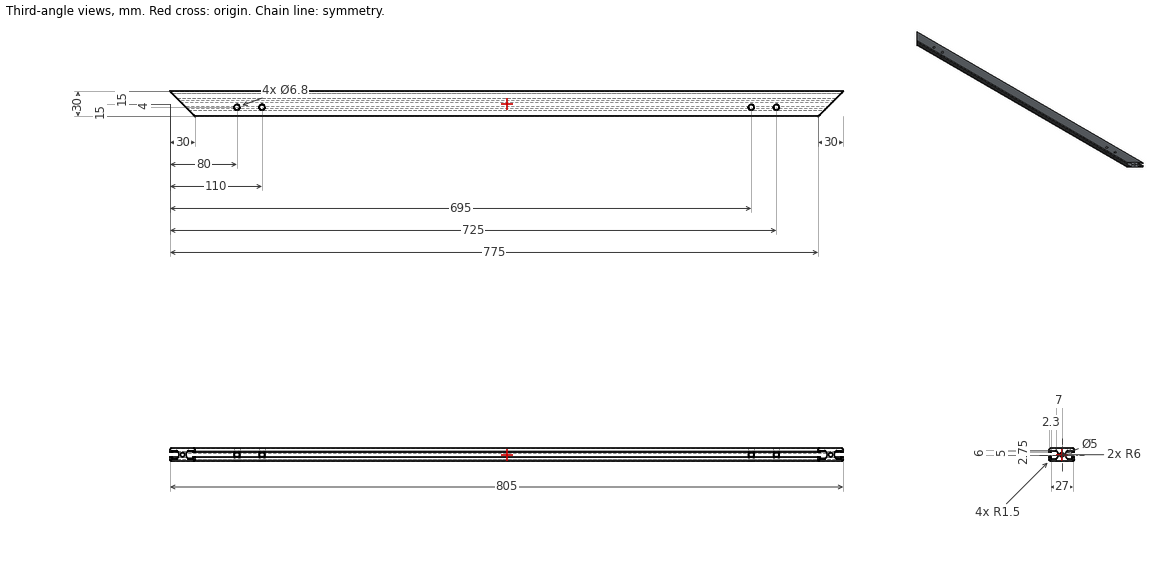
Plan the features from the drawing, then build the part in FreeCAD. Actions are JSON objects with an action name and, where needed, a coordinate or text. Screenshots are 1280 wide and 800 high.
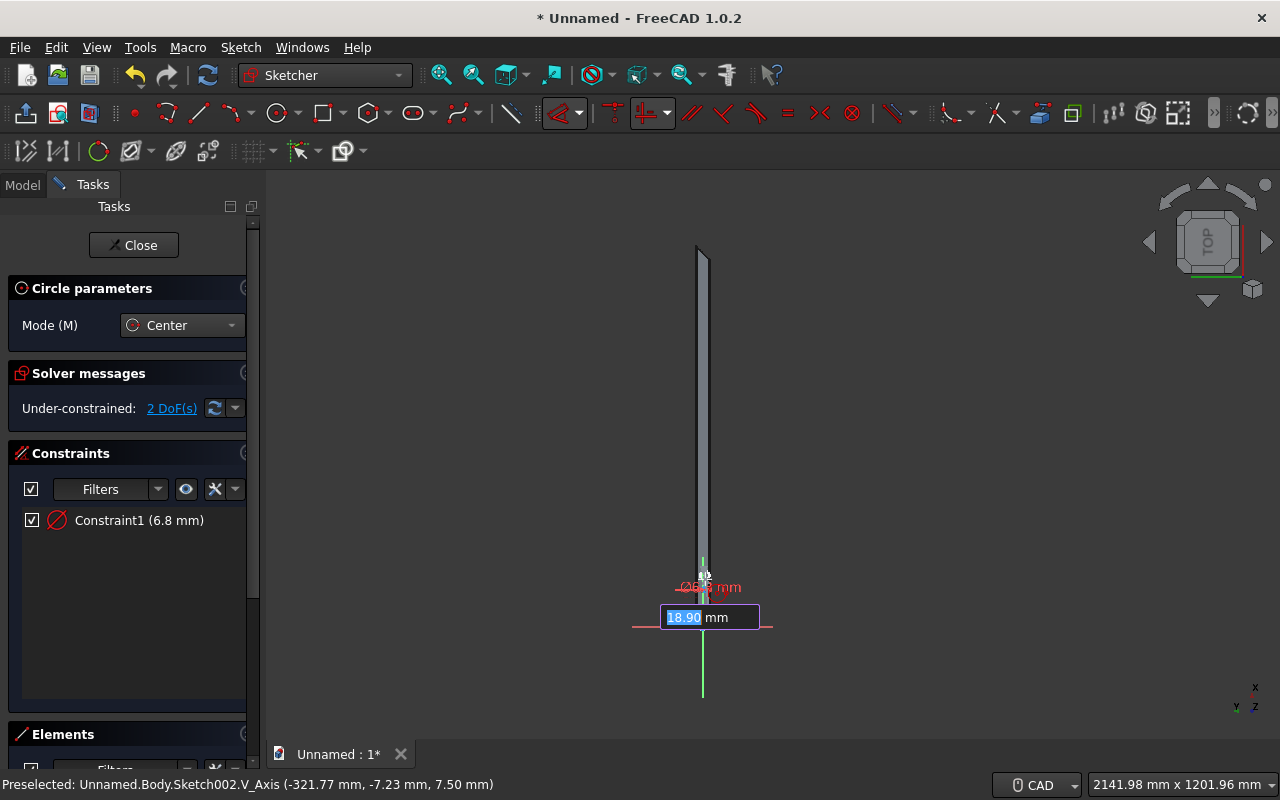
{"action": "scroll", "coordinate": [706, 574], "scroll_direction": "up", "scroll_amount": 9}
{"action": "mouse_move", "coordinate": [704, 571]}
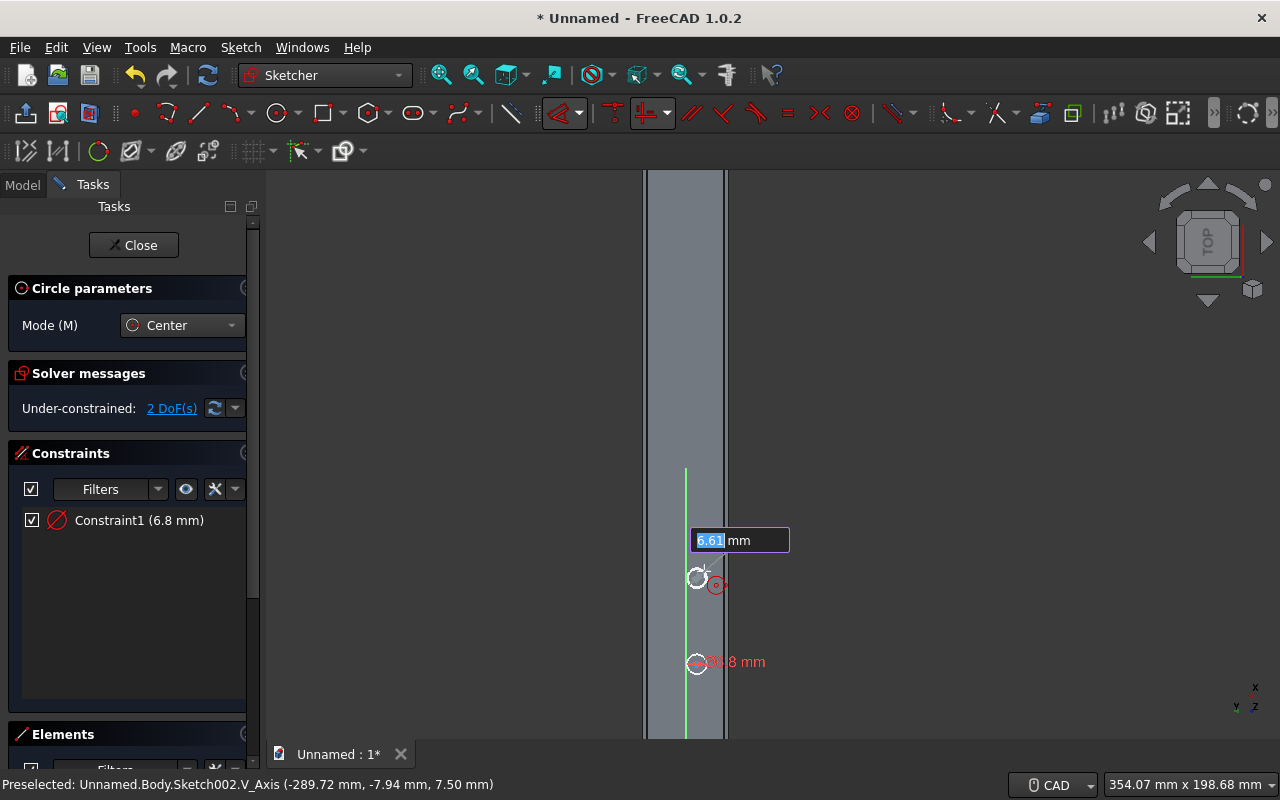
{"action": "type", "text": "6.8"}
{"action": "key", "text": "Return"}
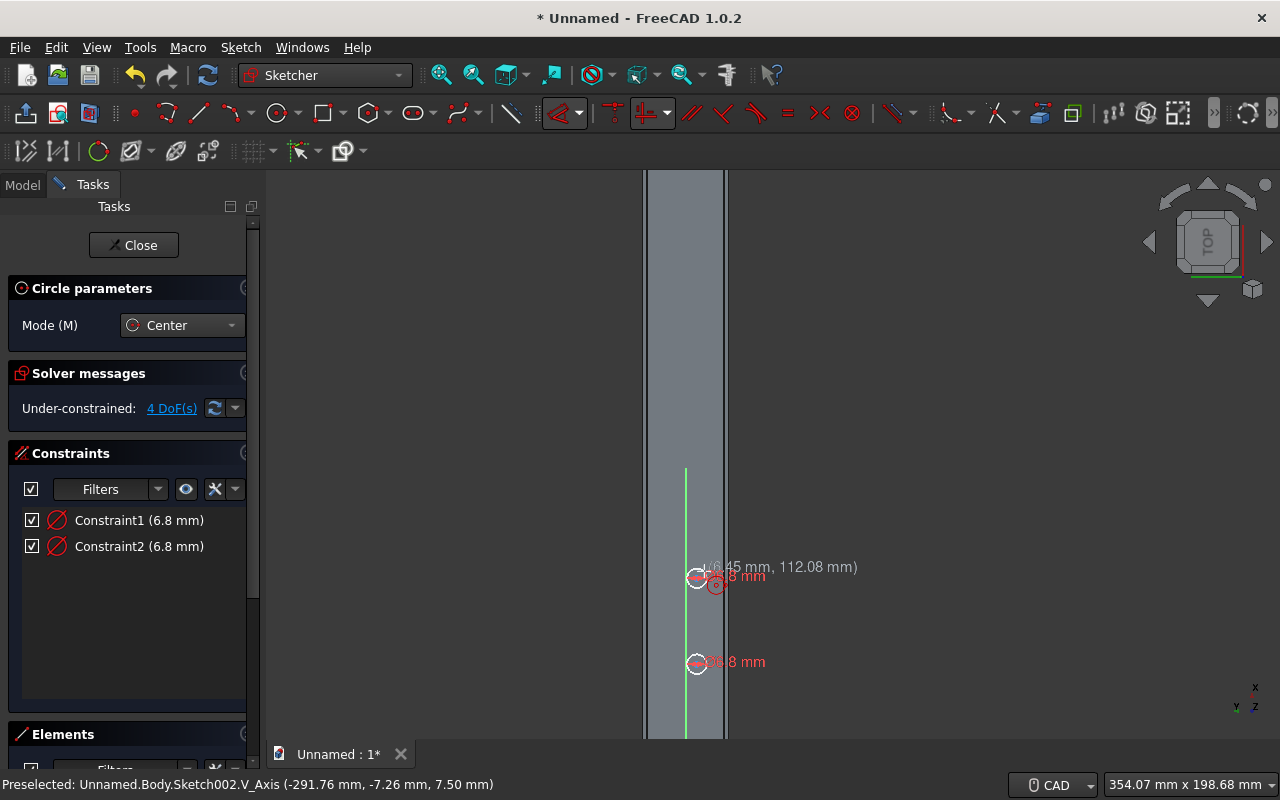
{"action": "scroll", "coordinate": [706, 574], "scroll_direction": "down", "scroll_amount": 9}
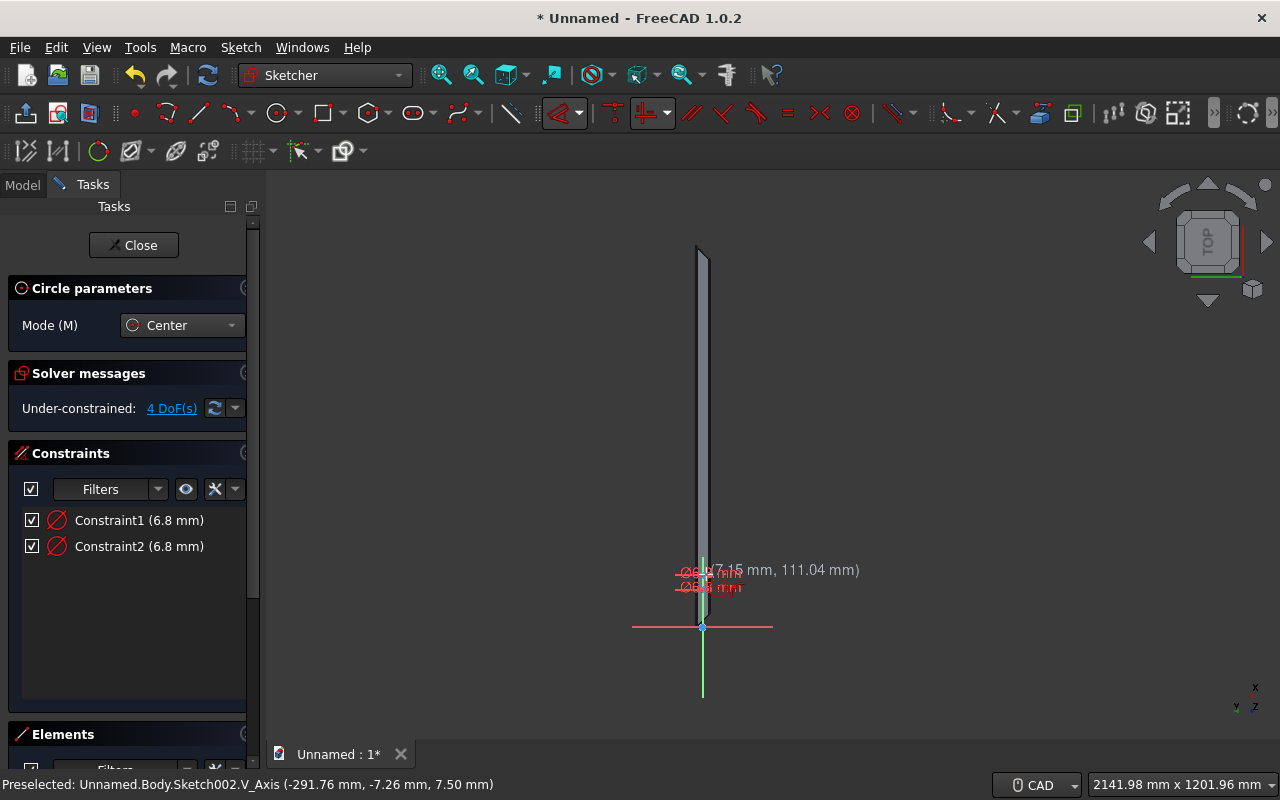
{"action": "scroll", "coordinate": [705, 298], "scroll_direction": "up", "scroll_amount": 14}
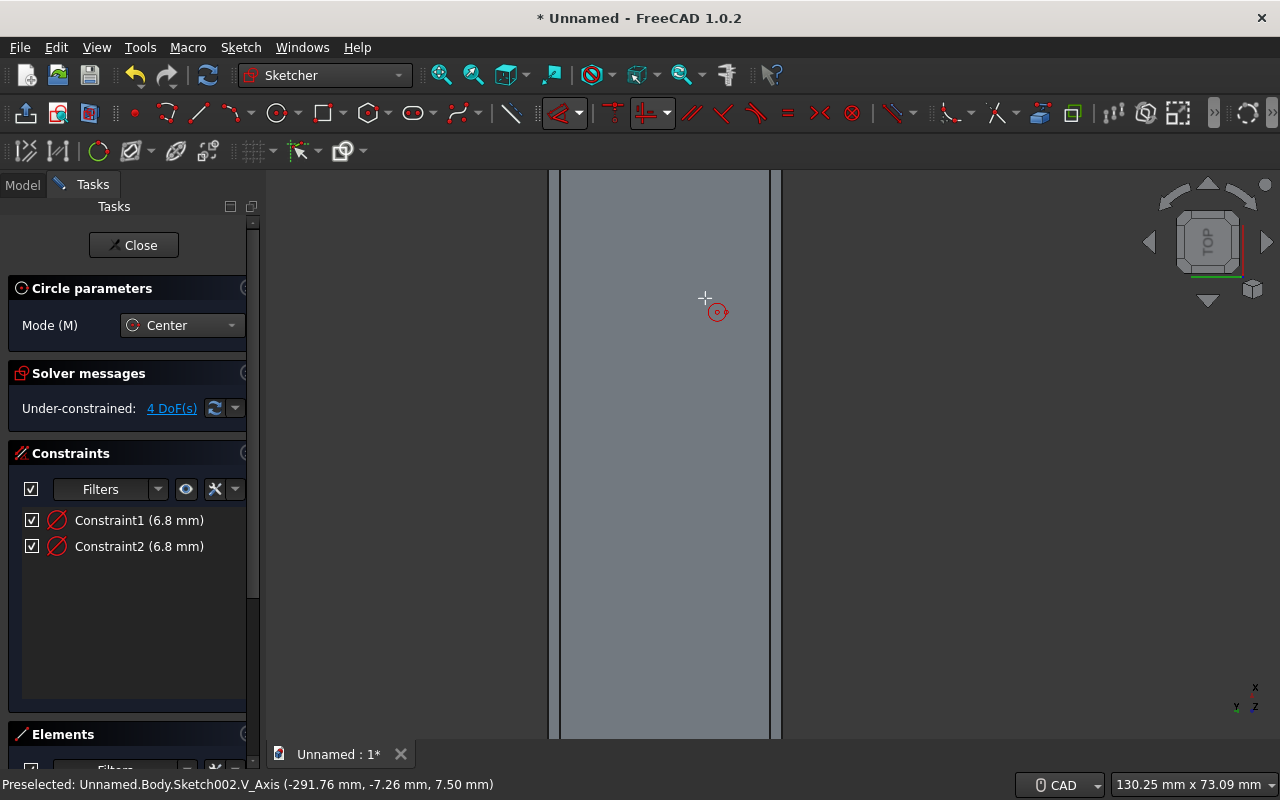
{"action": "left_click", "coordinate": [696, 300]}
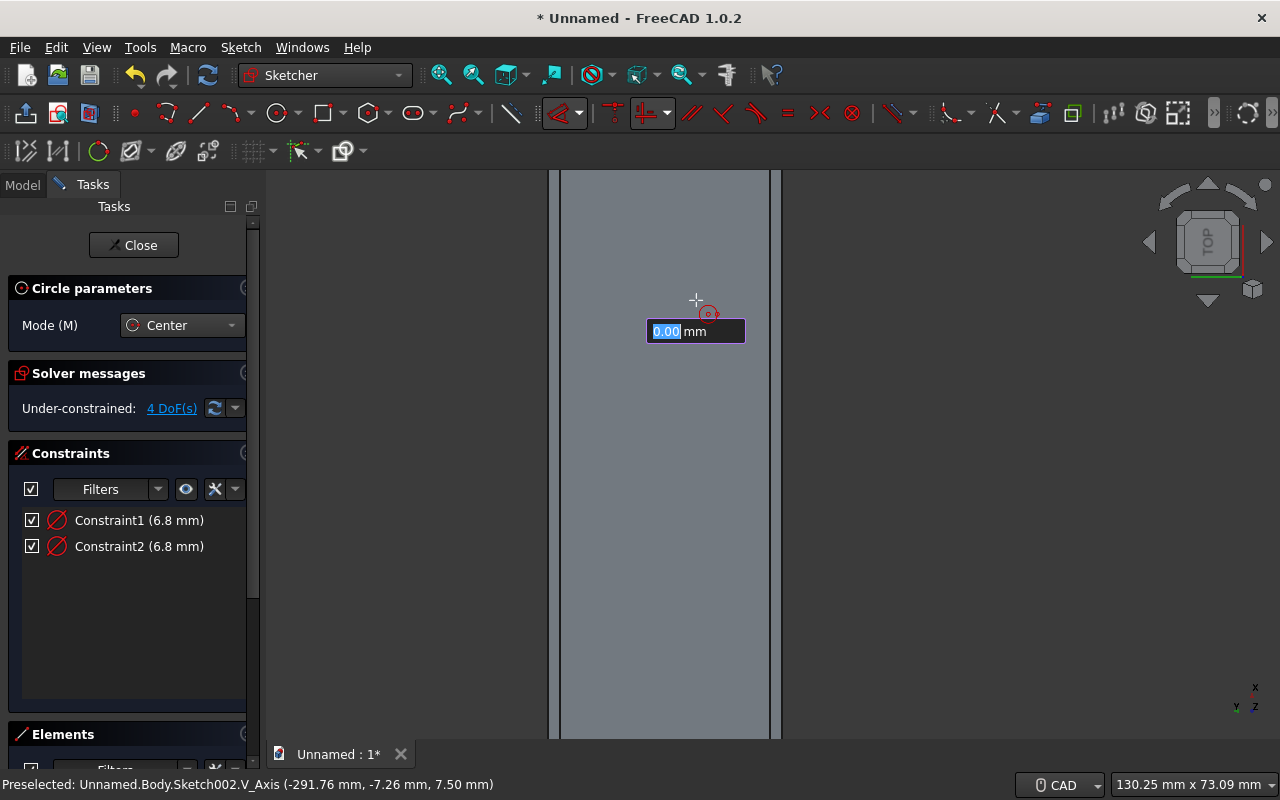
{"action": "scroll", "coordinate": [705, 298], "scroll_direction": "down", "scroll_amount": 14}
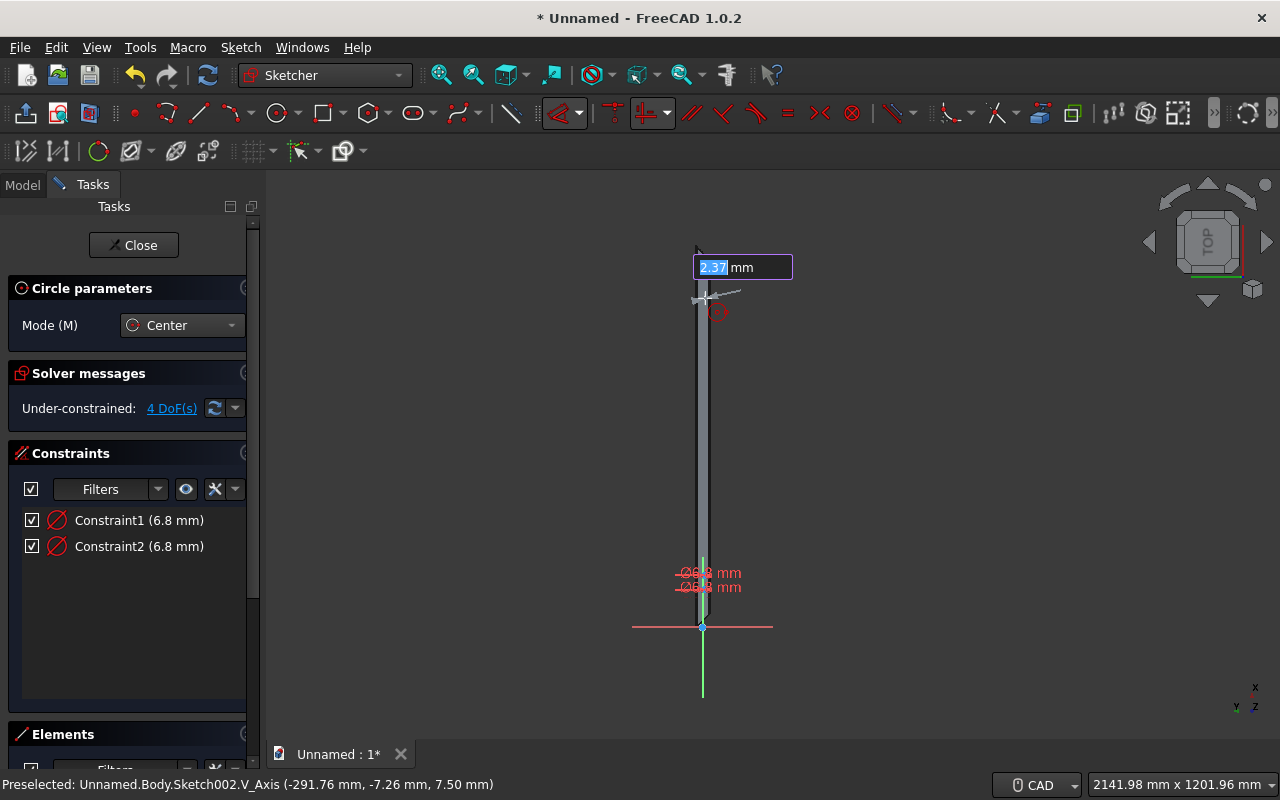
{"action": "scroll", "coordinate": [706, 297], "scroll_direction": "up", "scroll_amount": 9}
{"action": "mouse_move", "coordinate": [704, 297]}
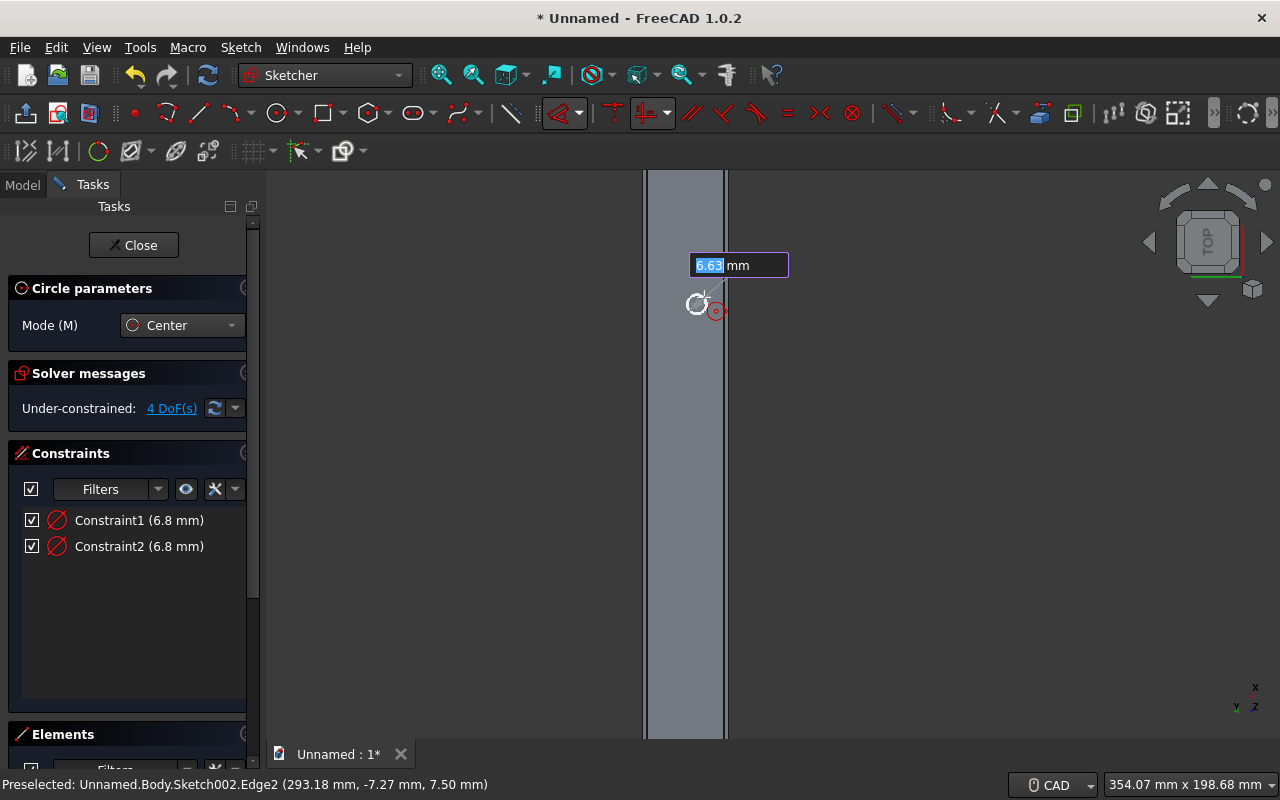
{"action": "type", "text": "6.8"}
{"action": "key", "text": "Return"}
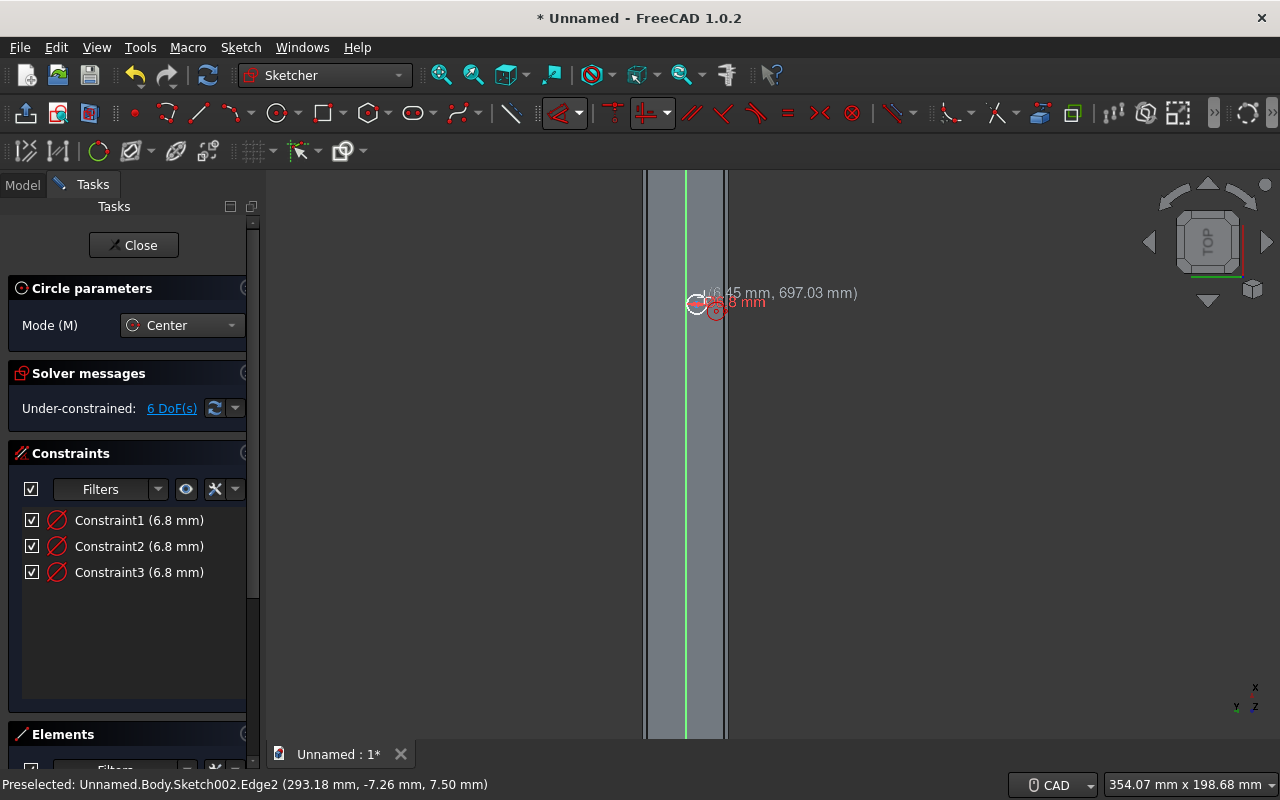
{"action": "scroll", "coordinate": [697, 218], "scroll_direction": "up", "scroll_amount": 5}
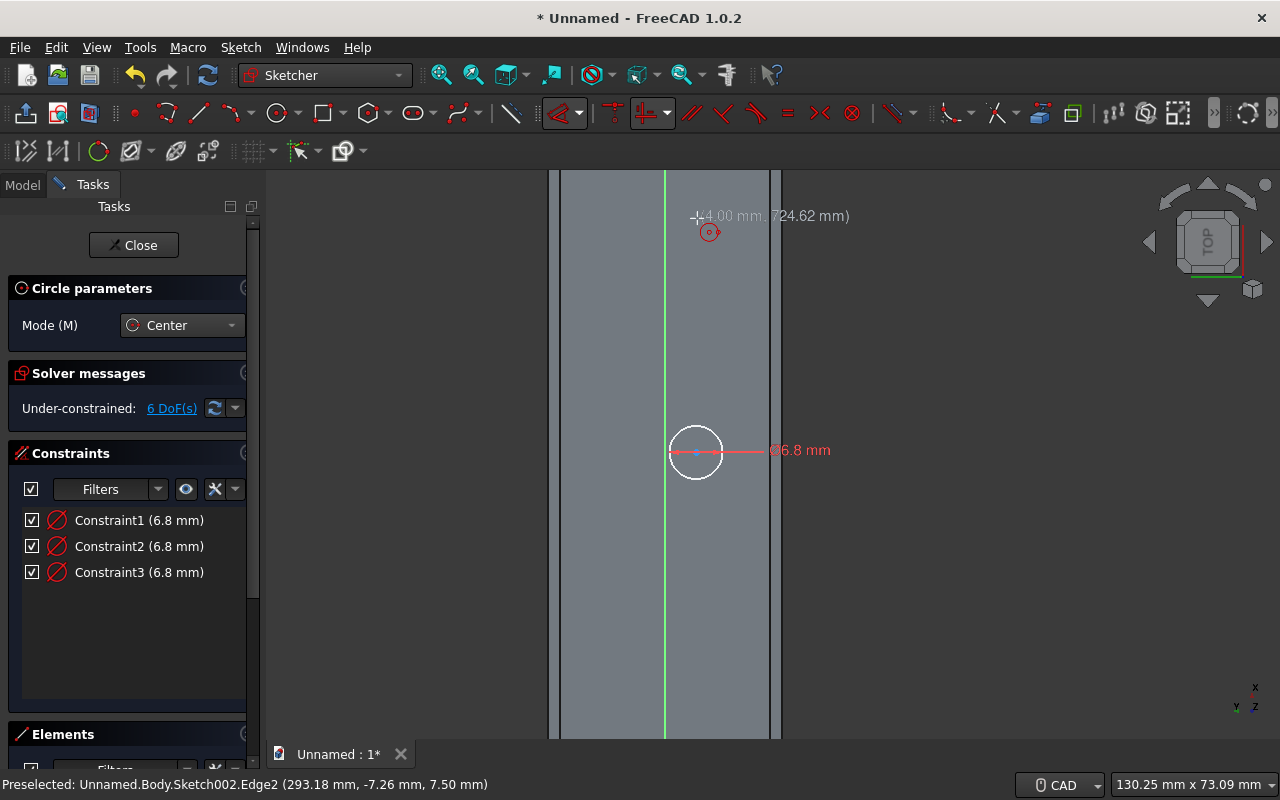
{"action": "left_click", "coordinate": [696, 218]}